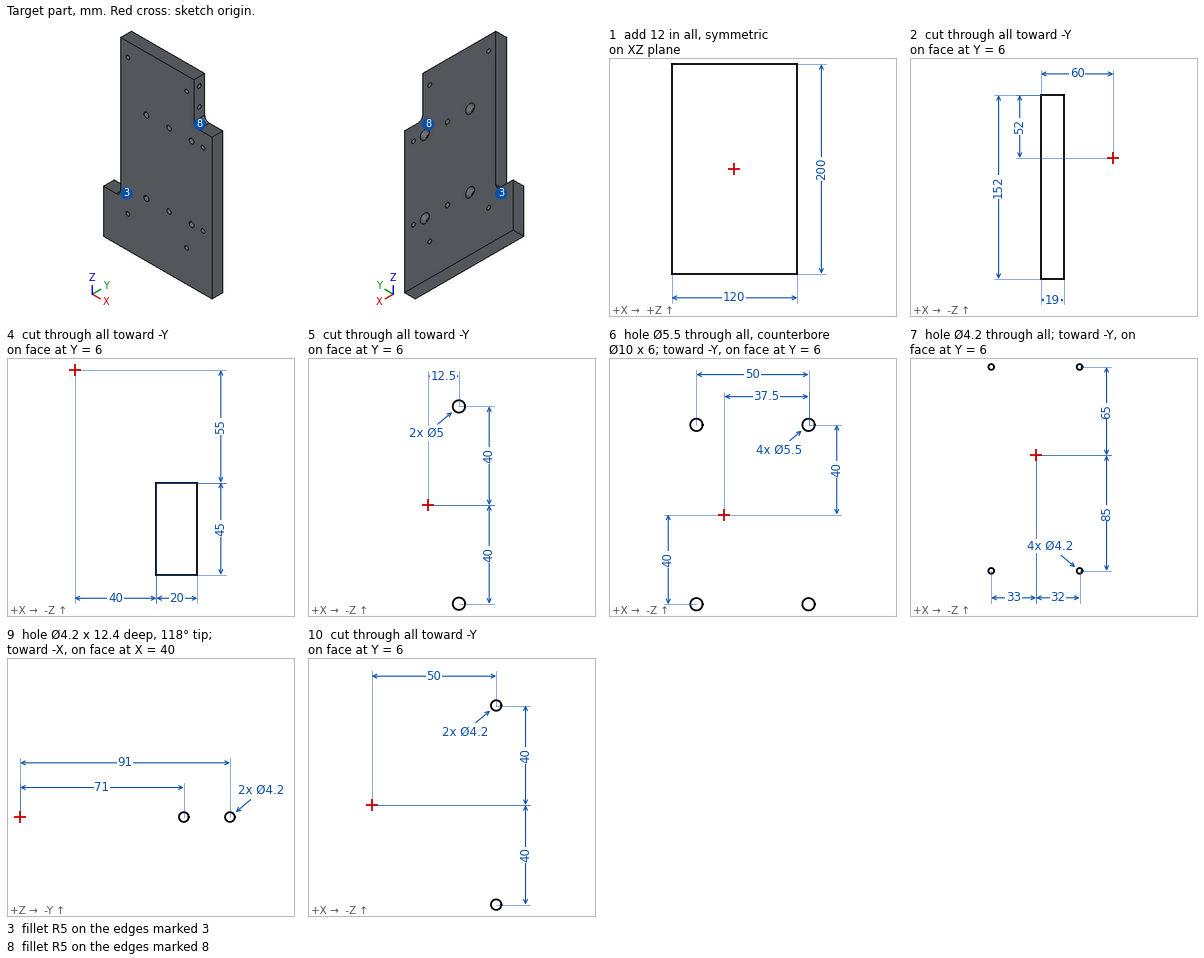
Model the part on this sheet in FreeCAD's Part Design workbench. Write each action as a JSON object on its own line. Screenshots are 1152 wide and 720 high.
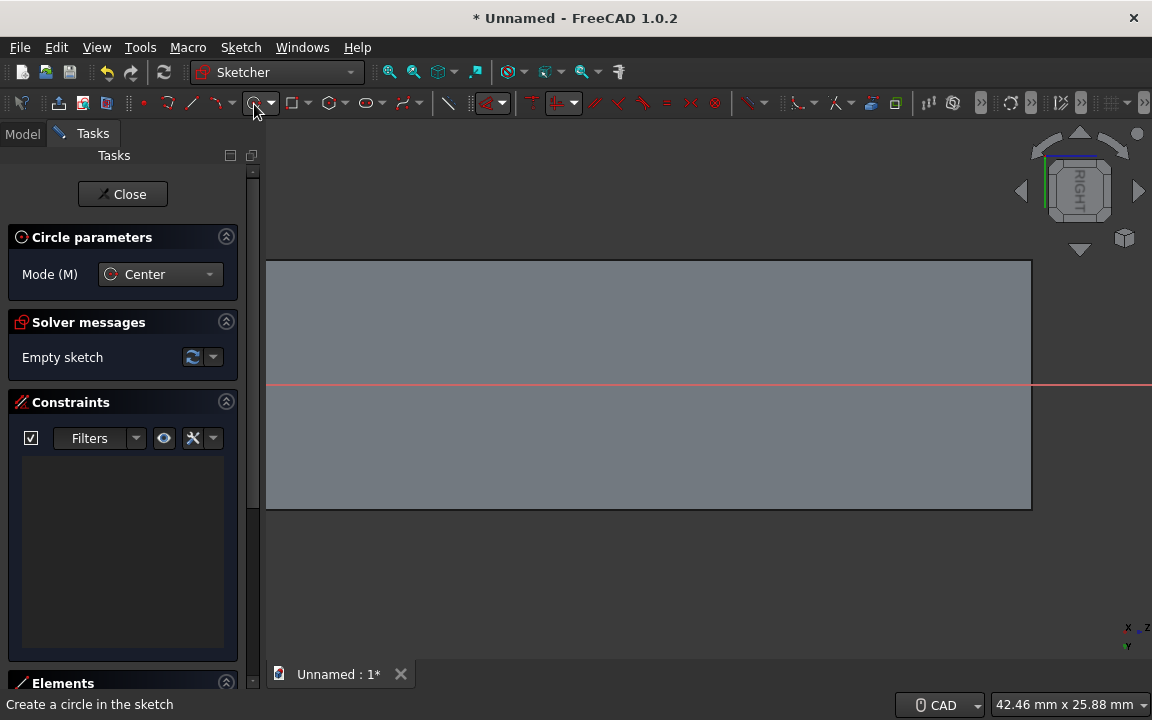
{"action": "left_click", "coordinate": [844, 385]}
{"action": "left_click", "coordinate": [875, 354]}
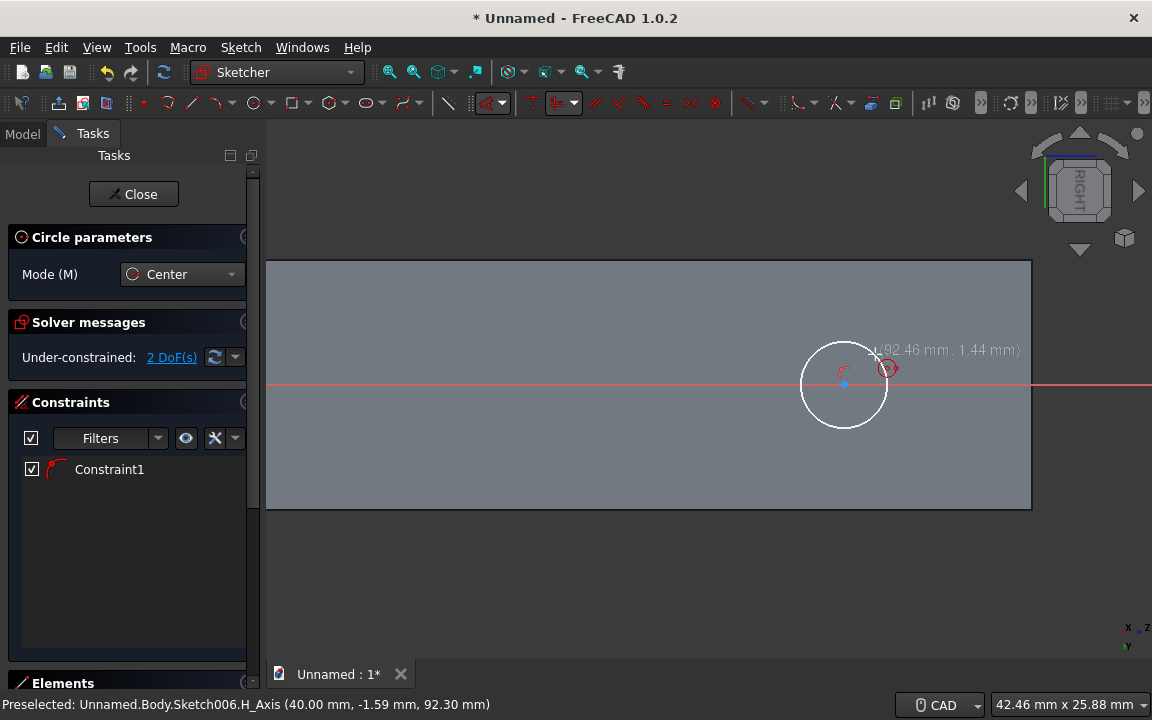
{"action": "left_click", "coordinate": [427, 385]}
{"action": "left_click", "coordinate": [458, 354]}
{"action": "key", "text": "Escape"}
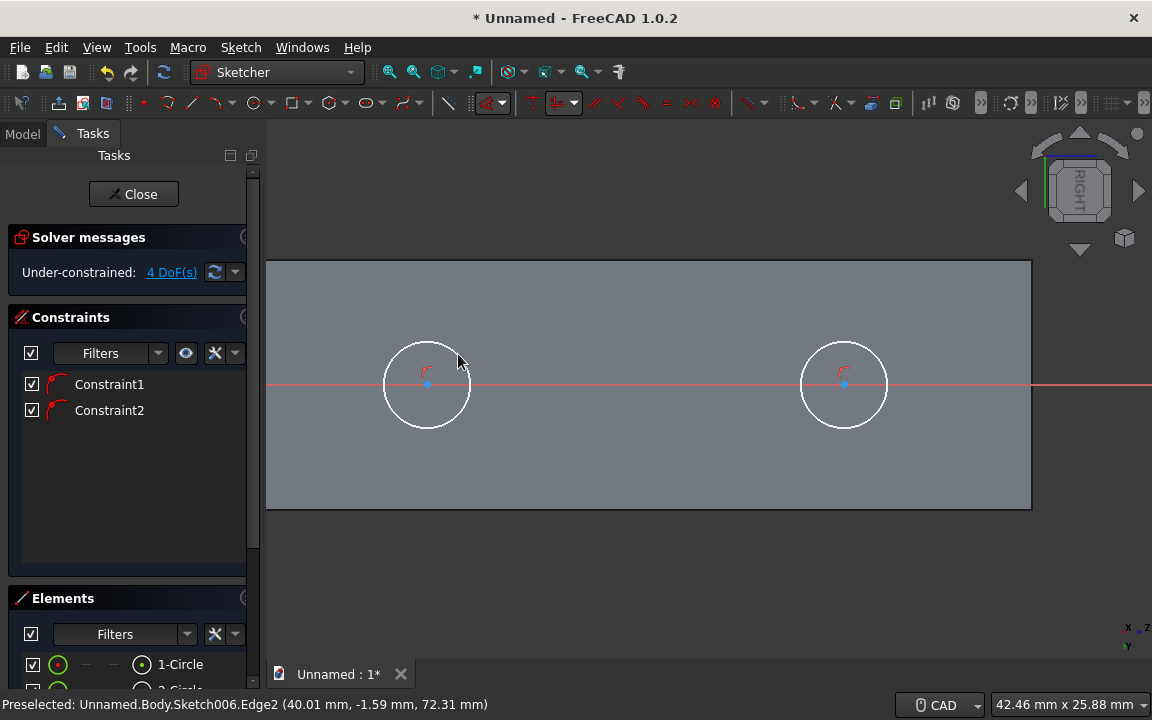
{"action": "left_click", "coordinate": [874, 354]}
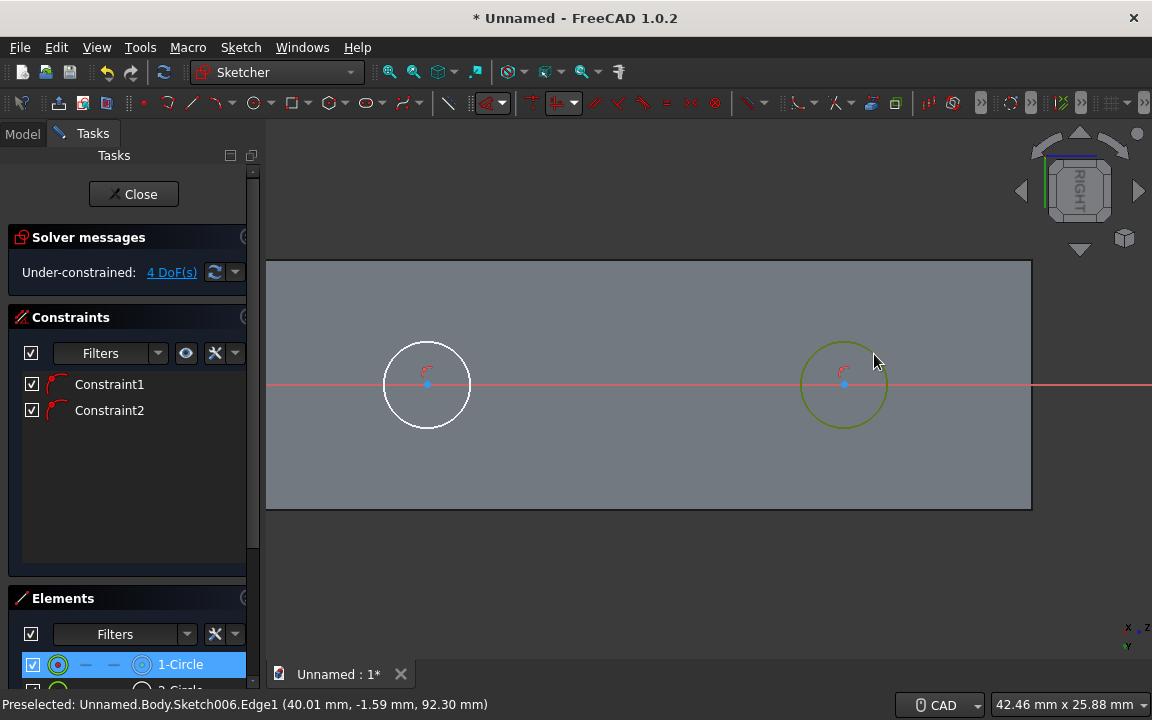
{"action": "left_click", "coordinate": [457, 354]}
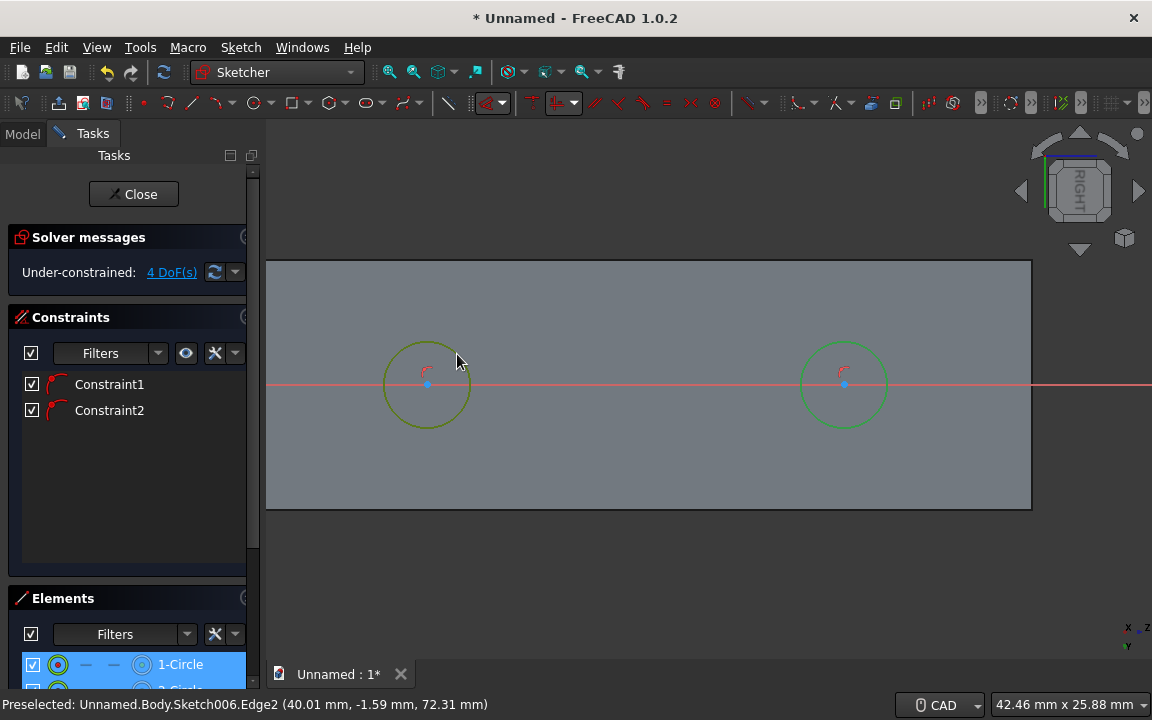
{"action": "left_click", "coordinate": [668, 104]}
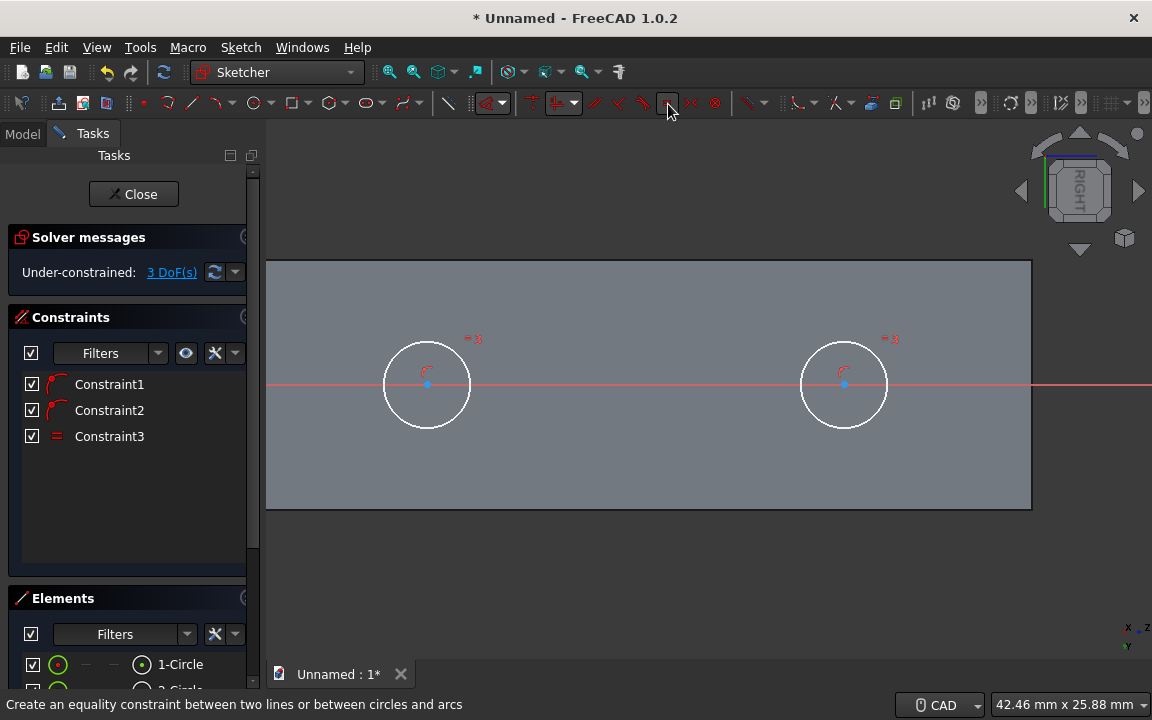
{"action": "left_click", "coordinate": [874, 354]}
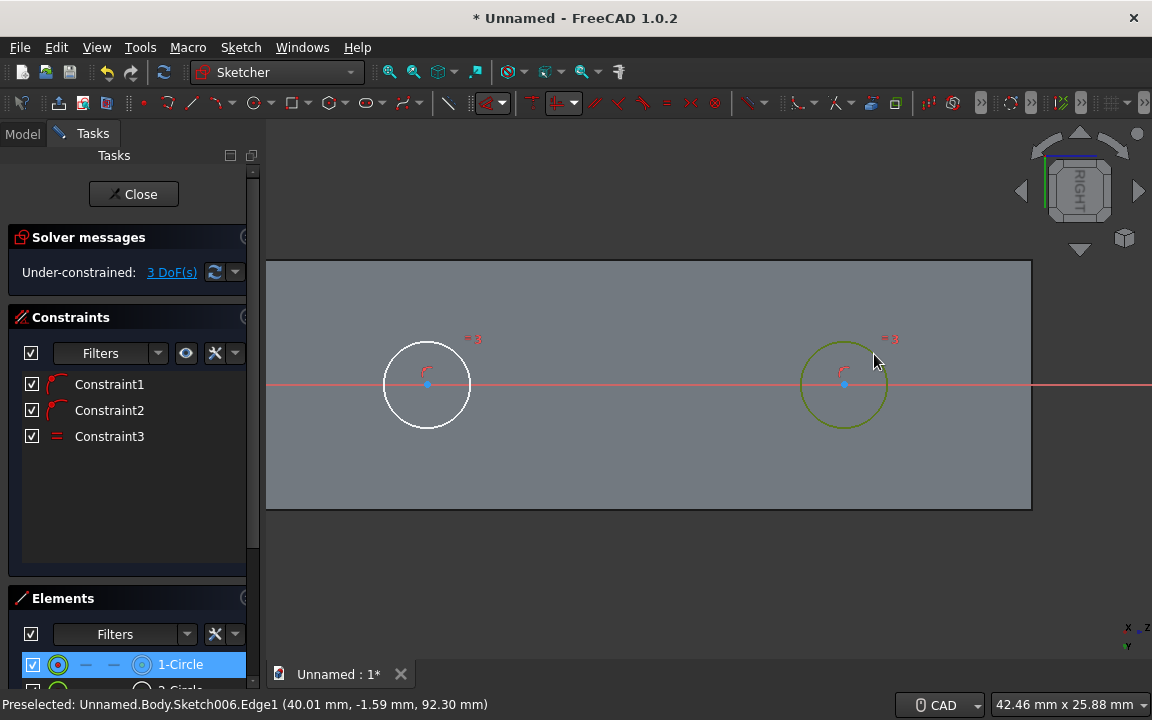
{"action": "key", "text": "k o"}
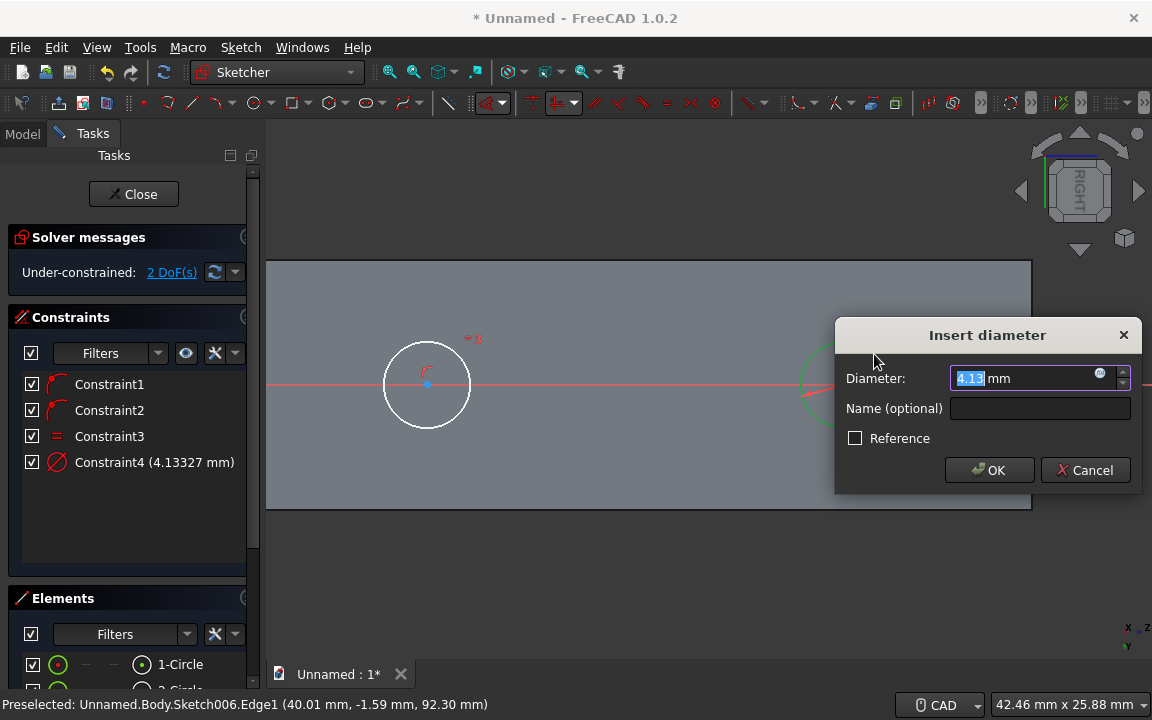
{"action": "type", "text": "4.2"}
{"action": "key", "text": "Return"}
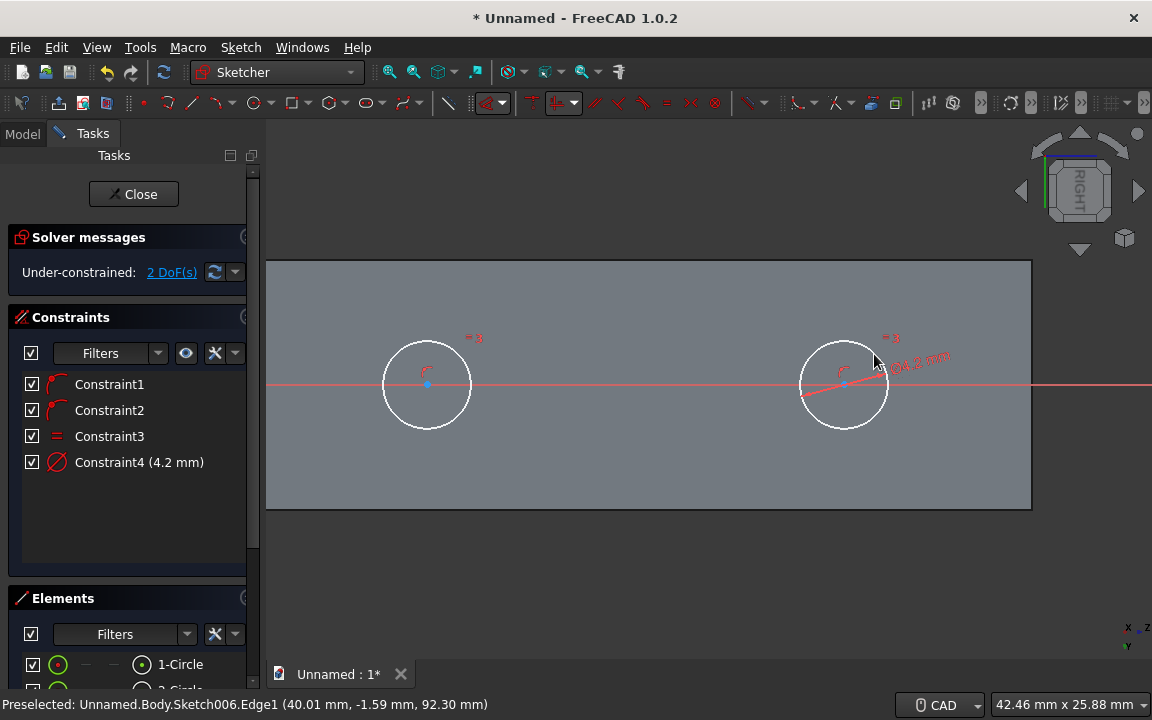
{"action": "left_click", "coordinate": [844, 385]}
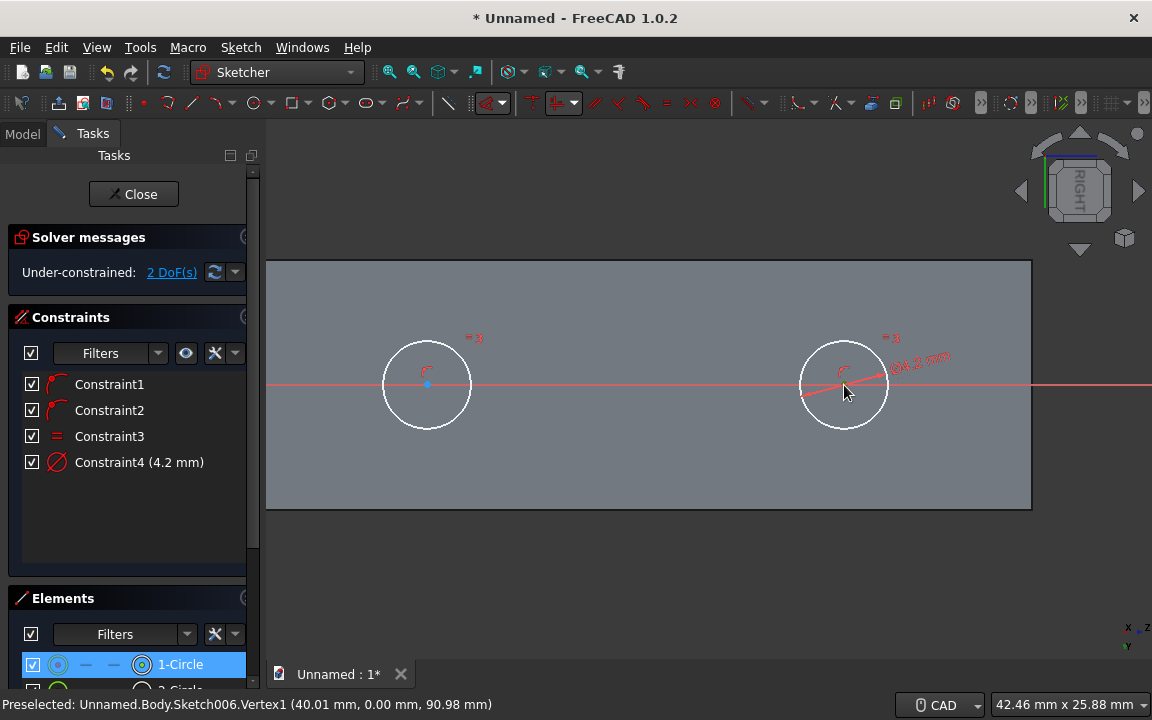
{"action": "left_click", "coordinate": [504, 104]}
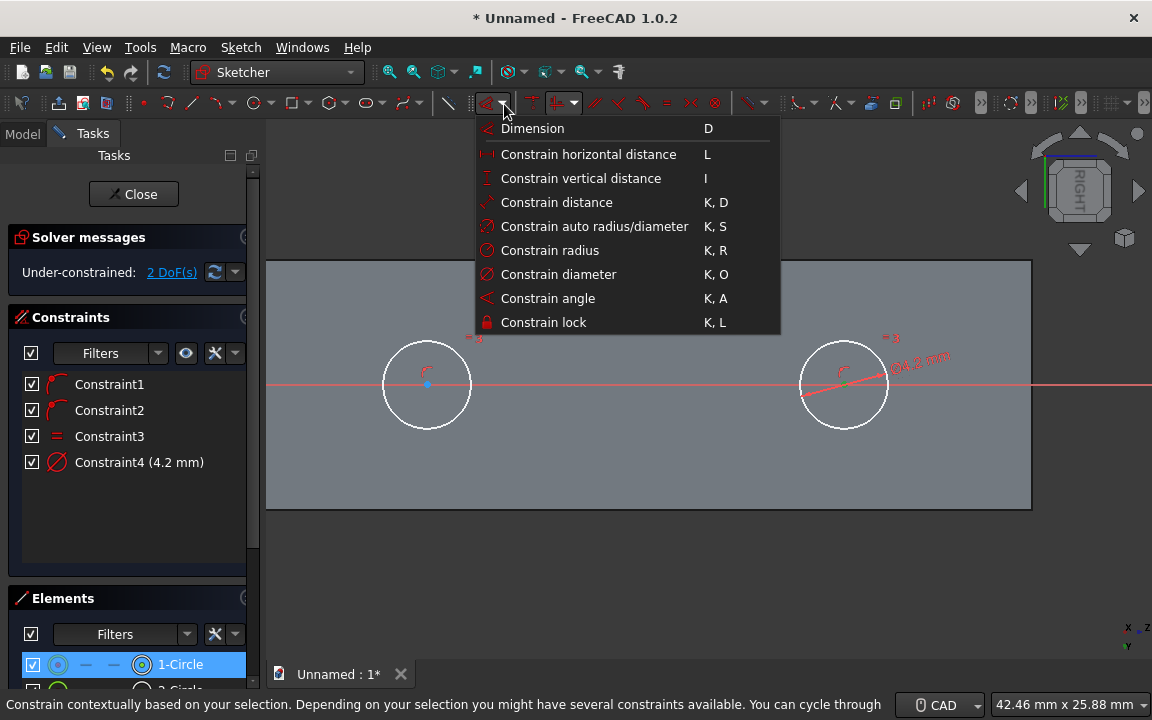
{"action": "left_click", "coordinate": [628, 154]}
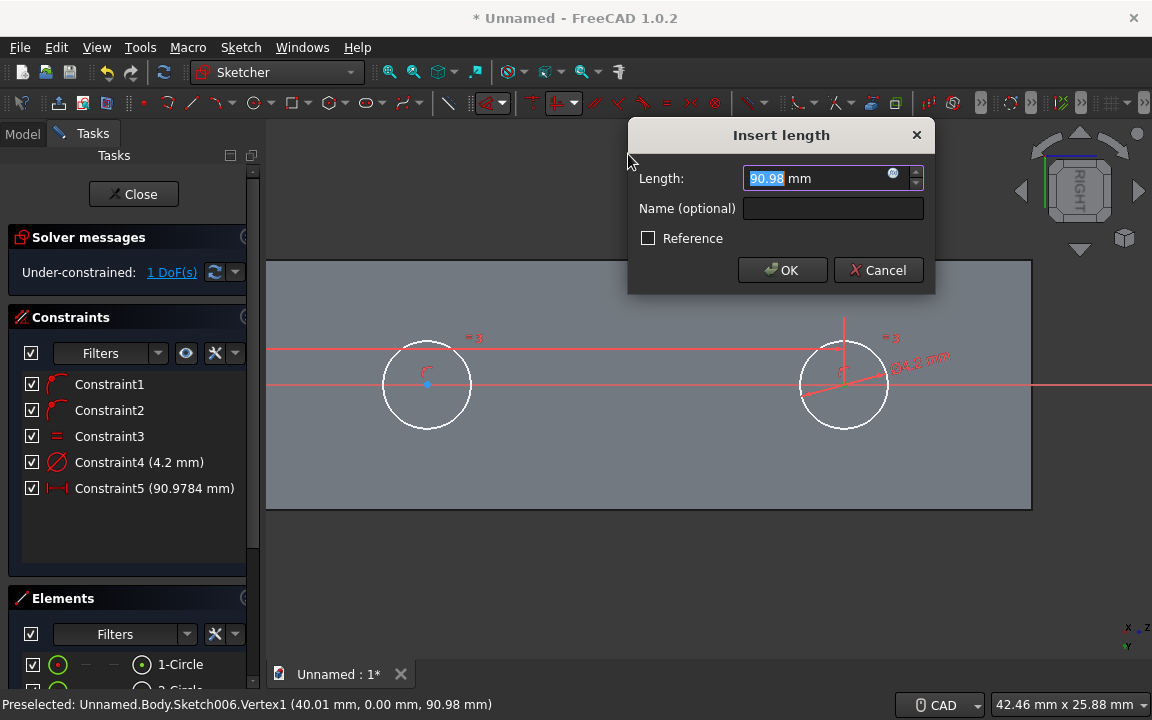
{"action": "type", "text": "91"}
{"action": "key", "text": "Return"}